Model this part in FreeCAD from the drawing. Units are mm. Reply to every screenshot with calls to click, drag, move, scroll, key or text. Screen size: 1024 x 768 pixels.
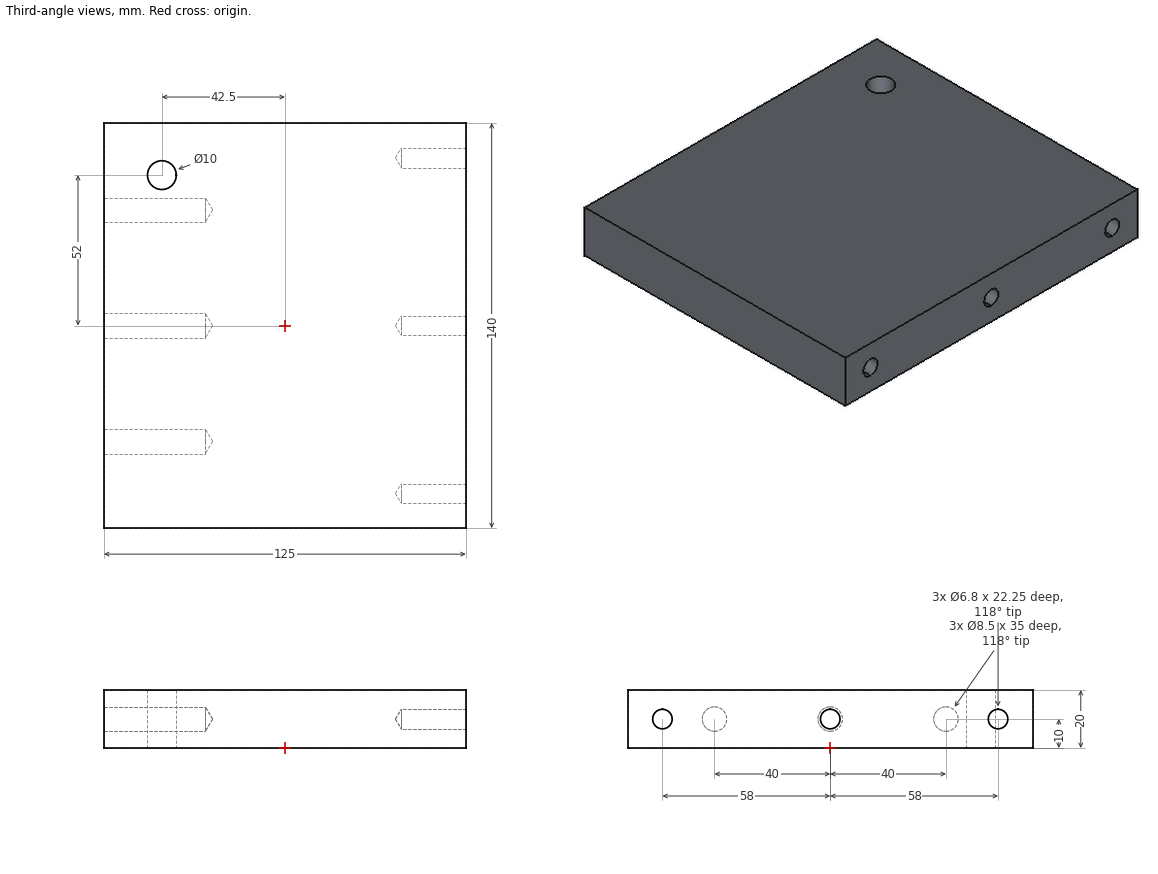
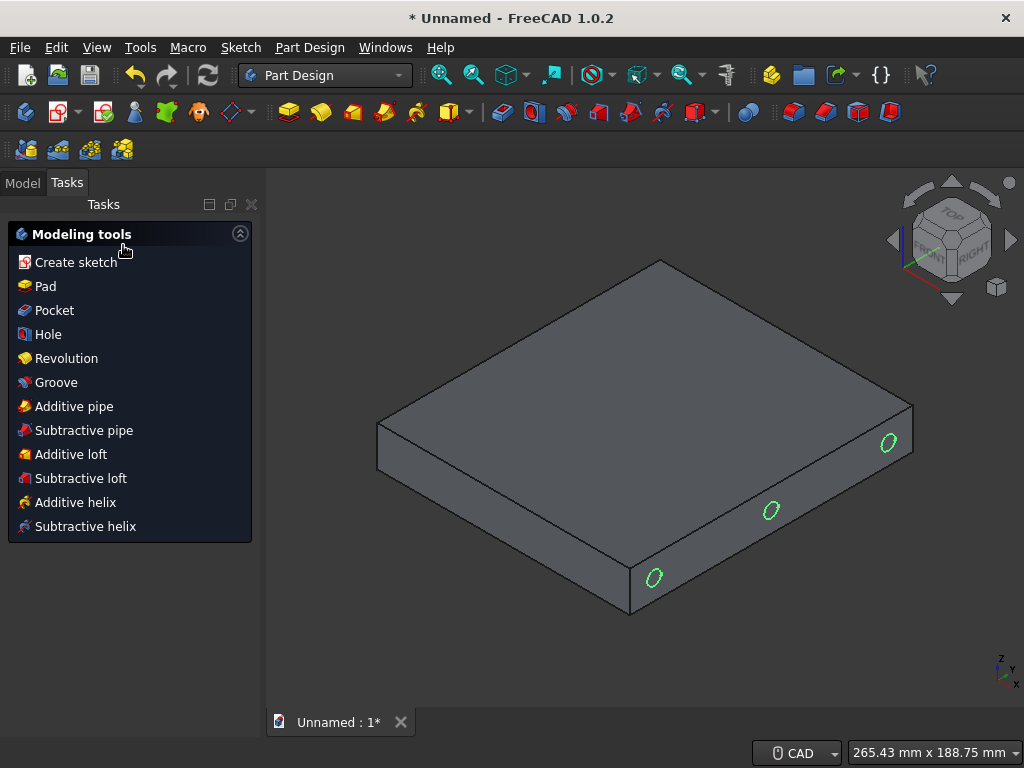
click(536, 112)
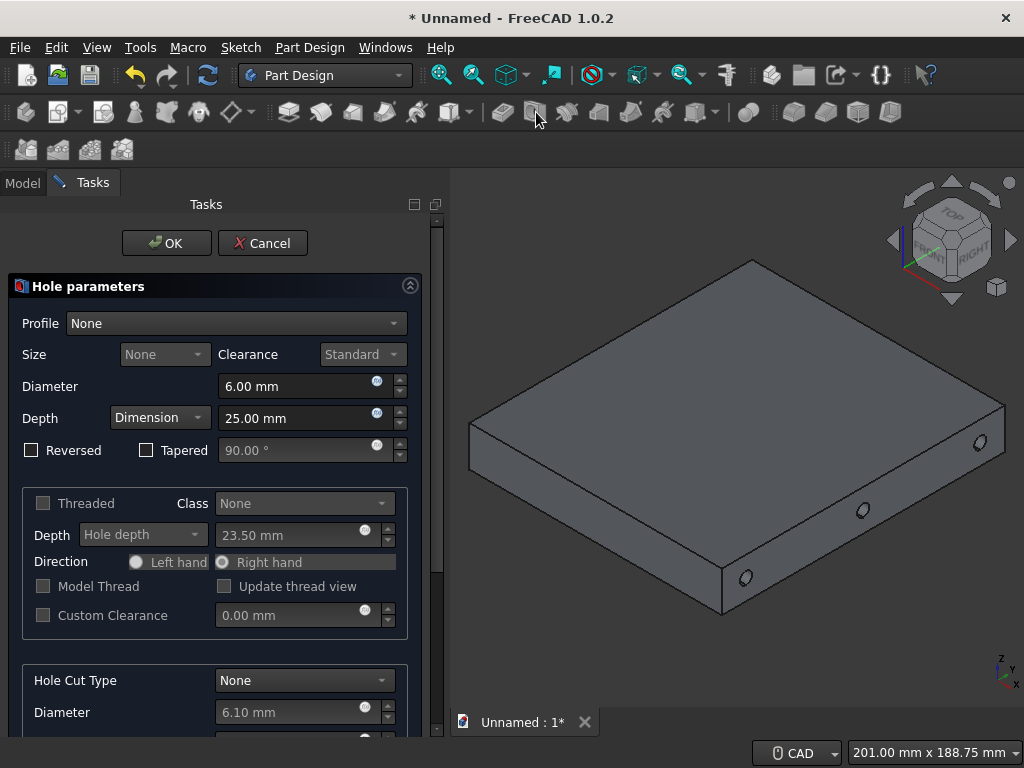
triple_click(305, 386)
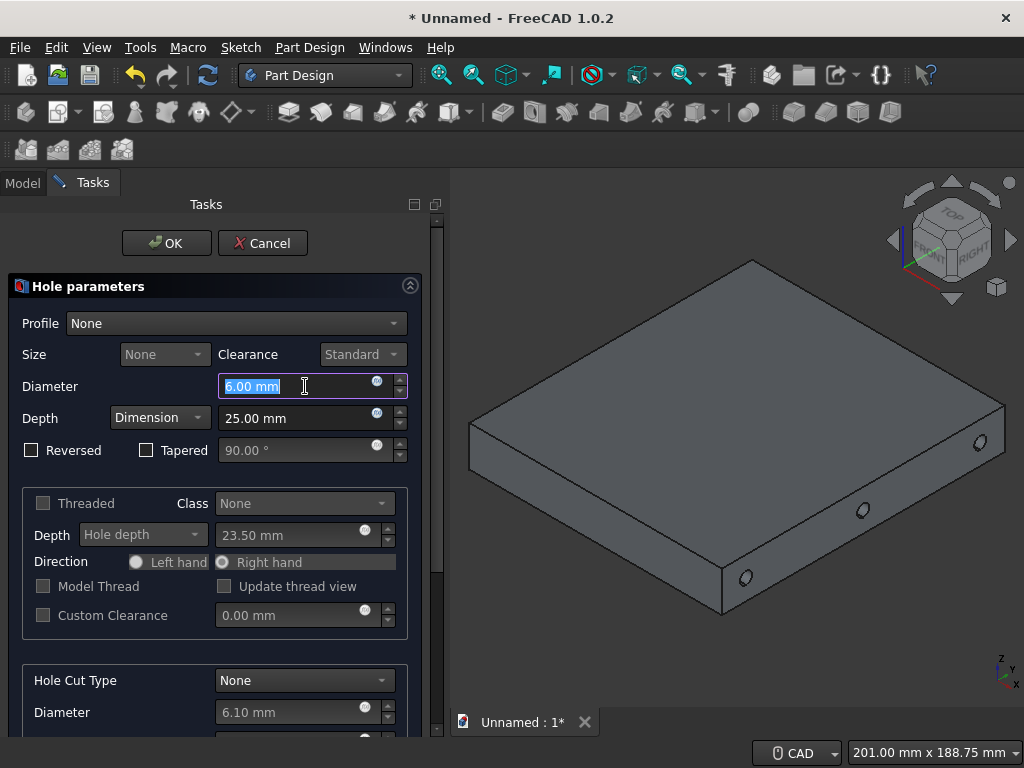
text(6.8)
key(Tab)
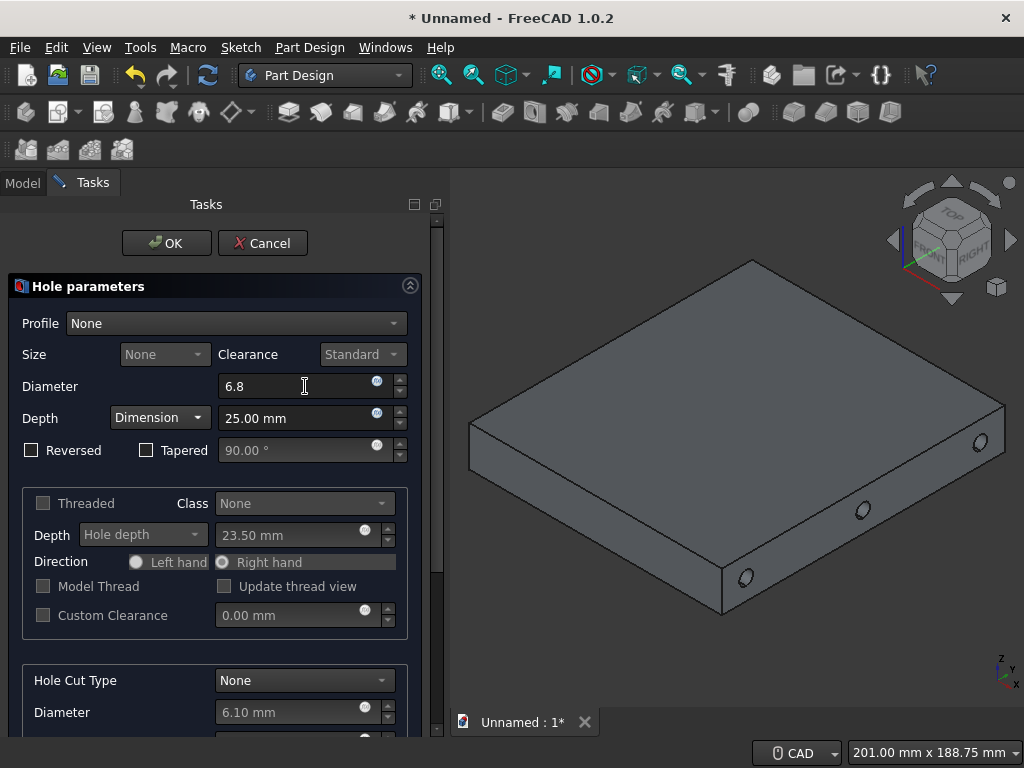
triple_click(305, 418)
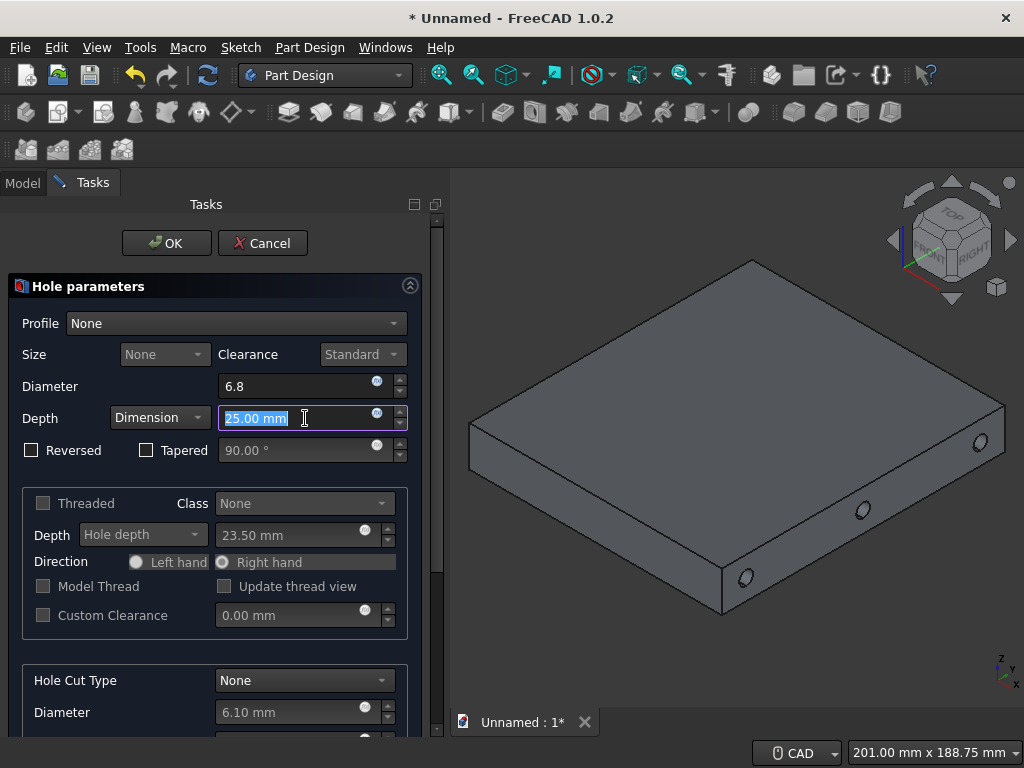
text(22.25)
key(Tab)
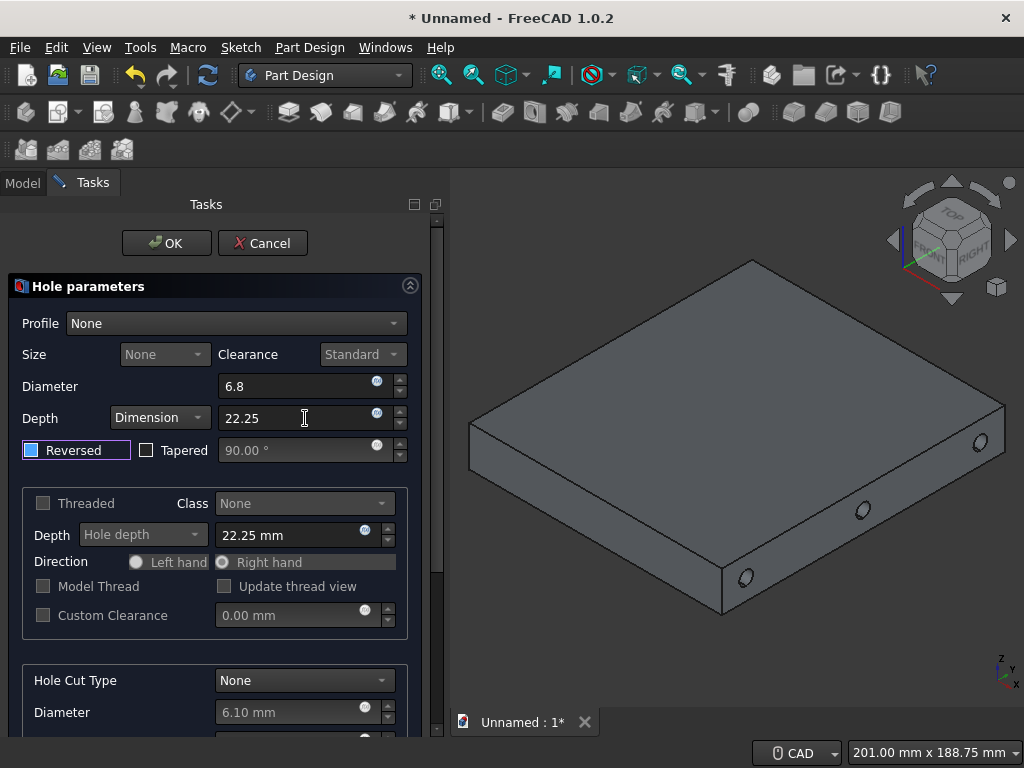
click(167, 243)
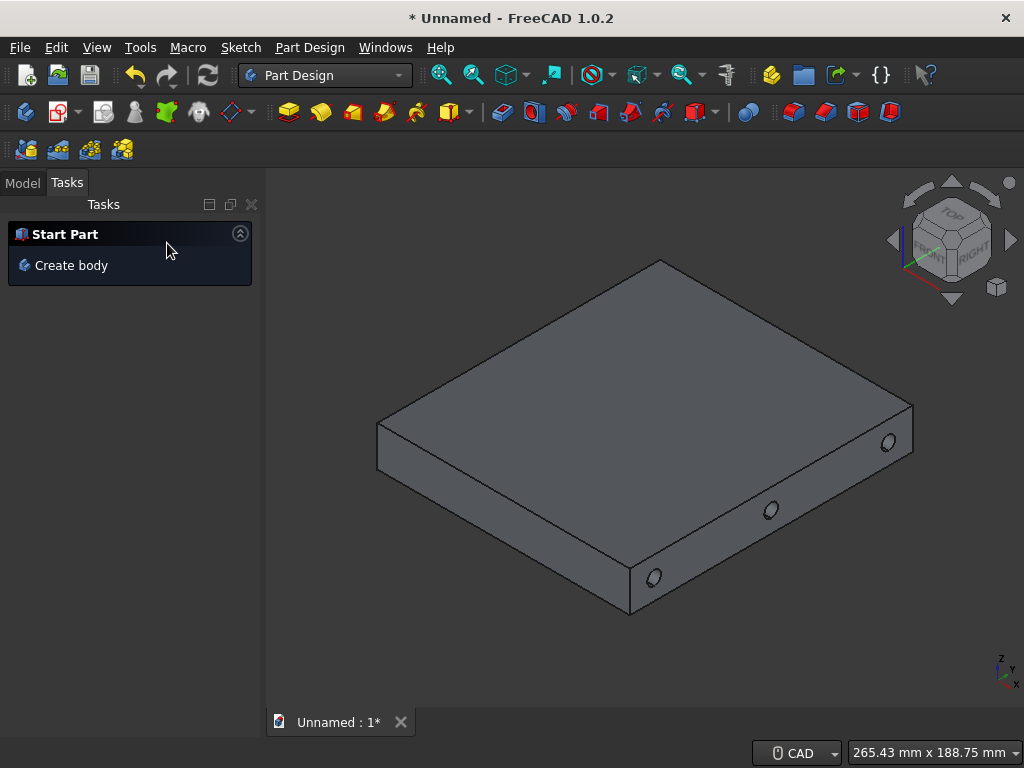
click(645, 413)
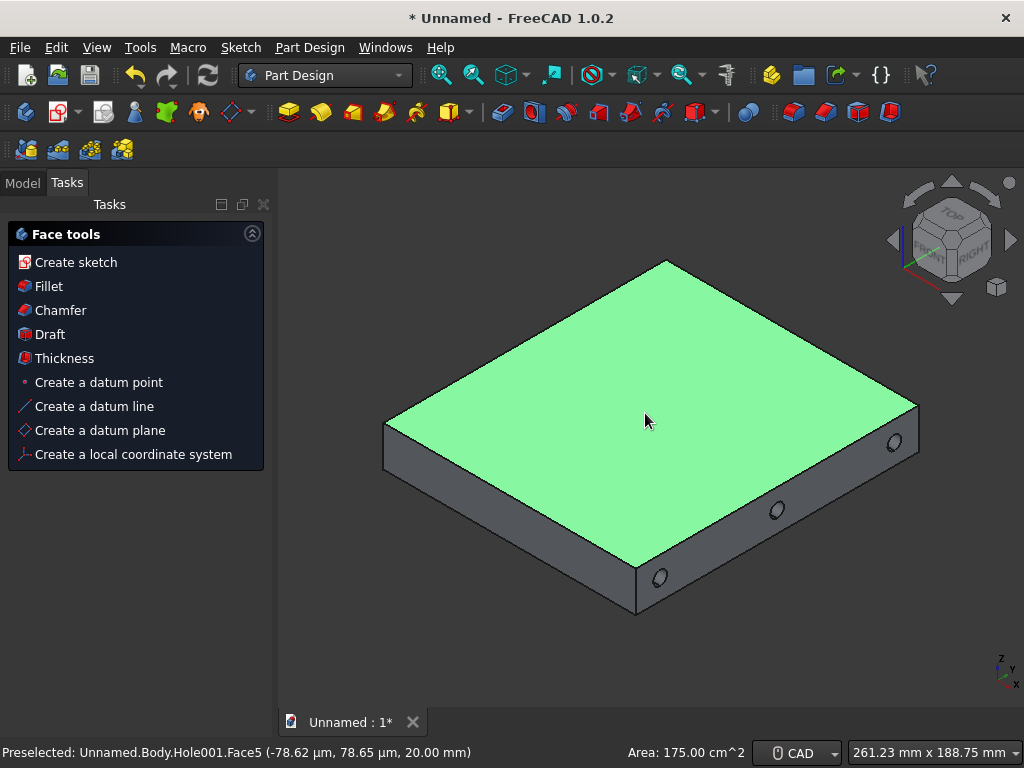
click(58, 112)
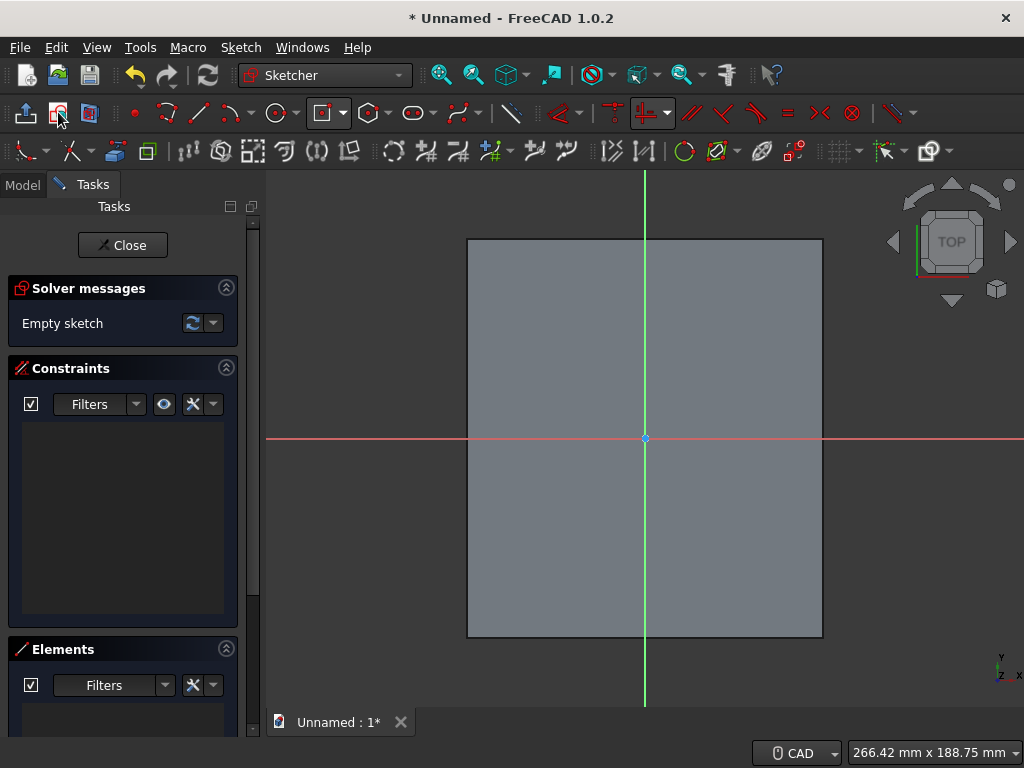
scroll(519, 276, up, 12)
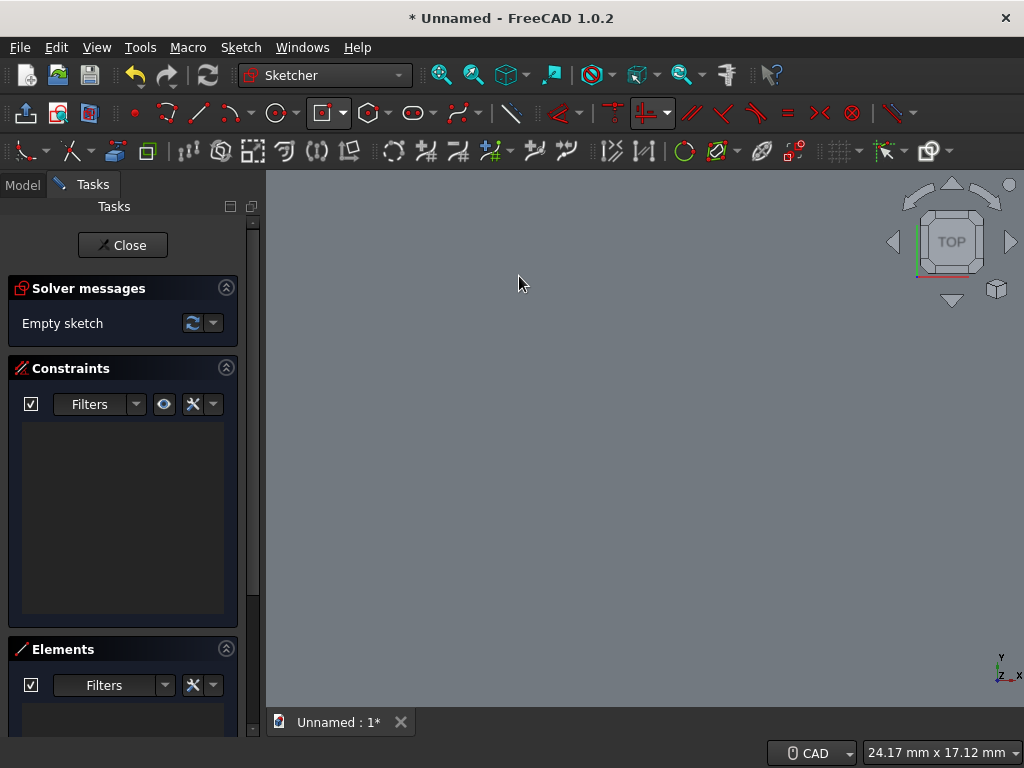
click(276, 114)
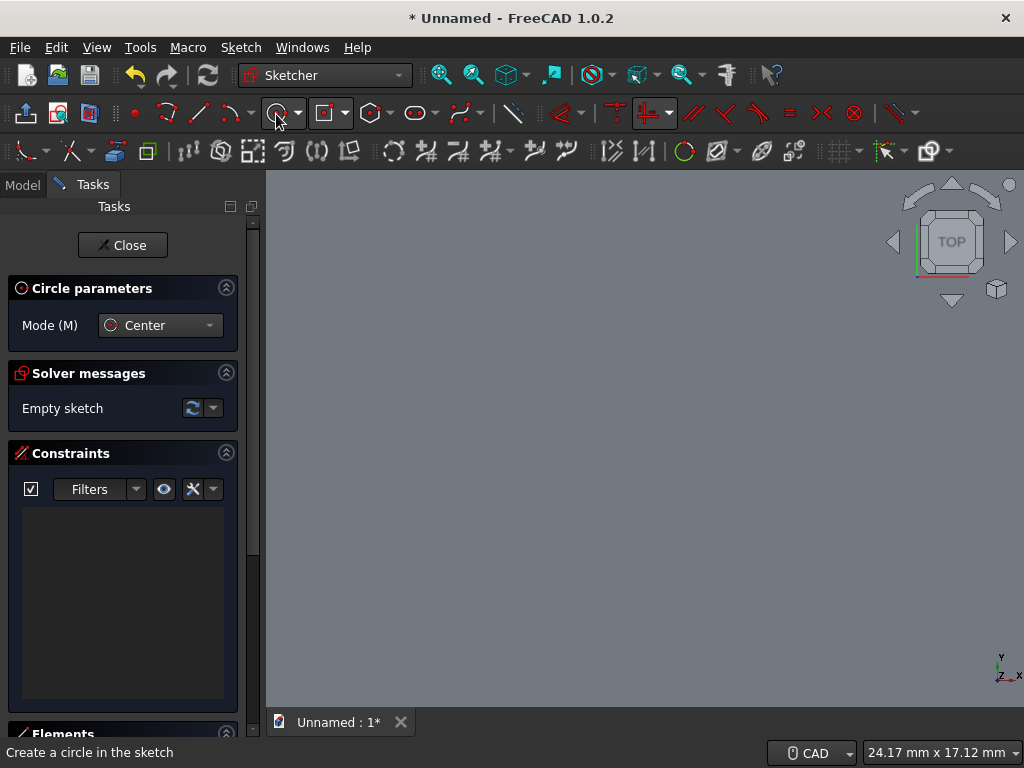
click(572, 434)
click(683, 324)
key(Escape)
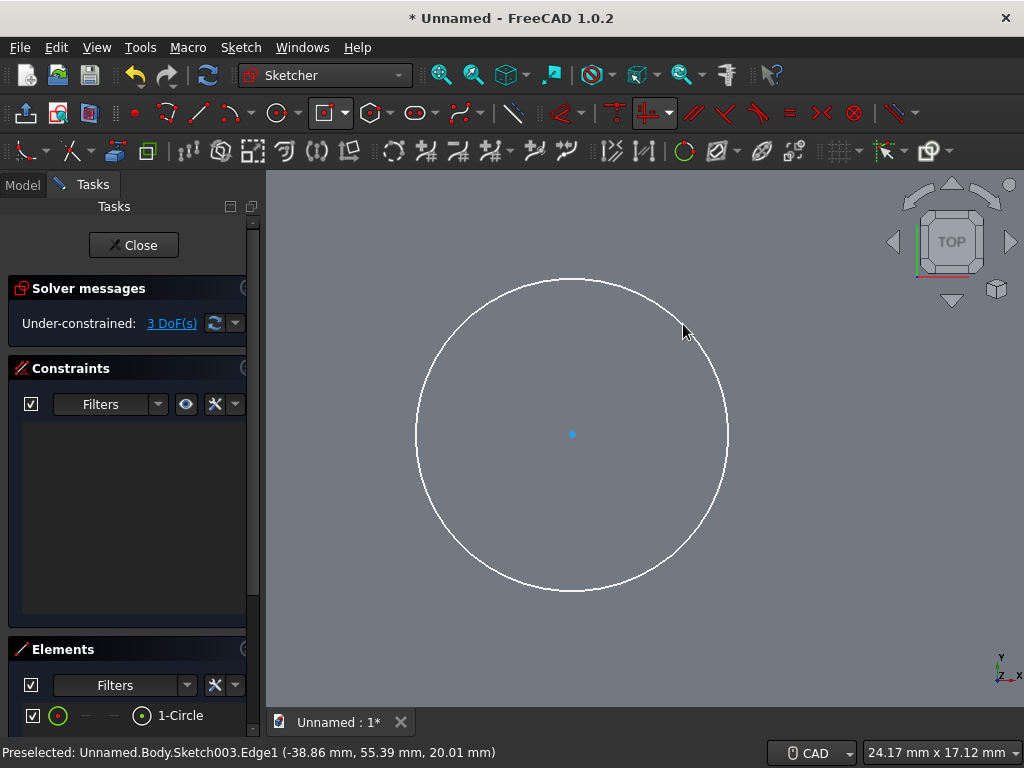
click(560, 114)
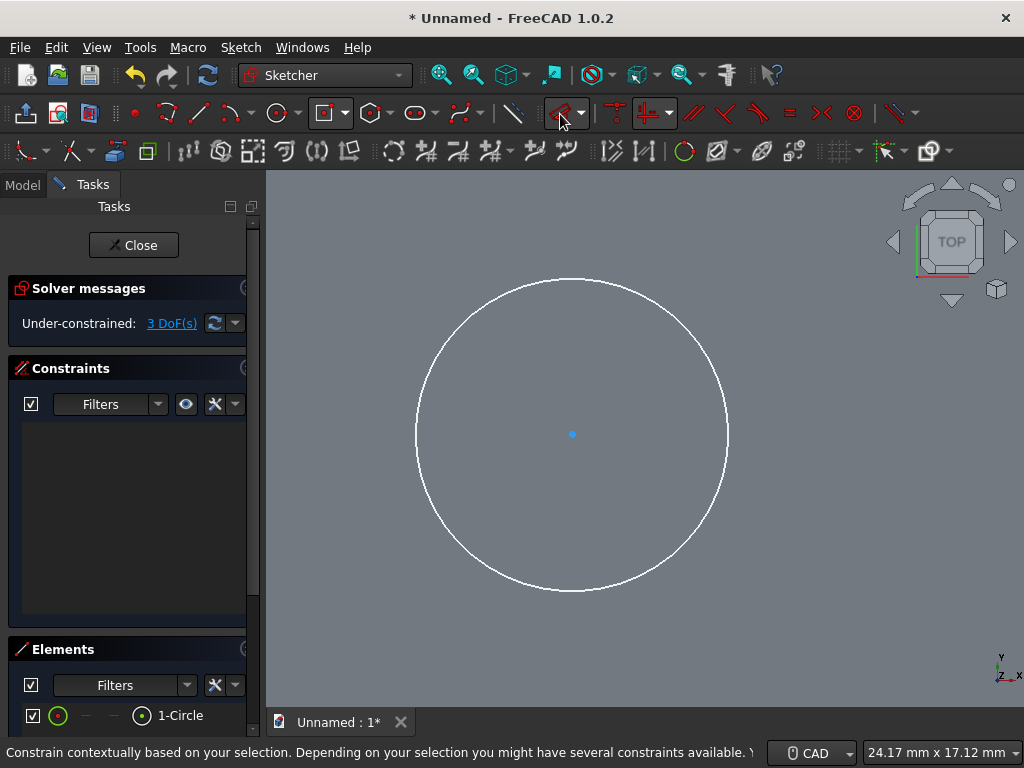
click(682, 324)
click(705, 301)